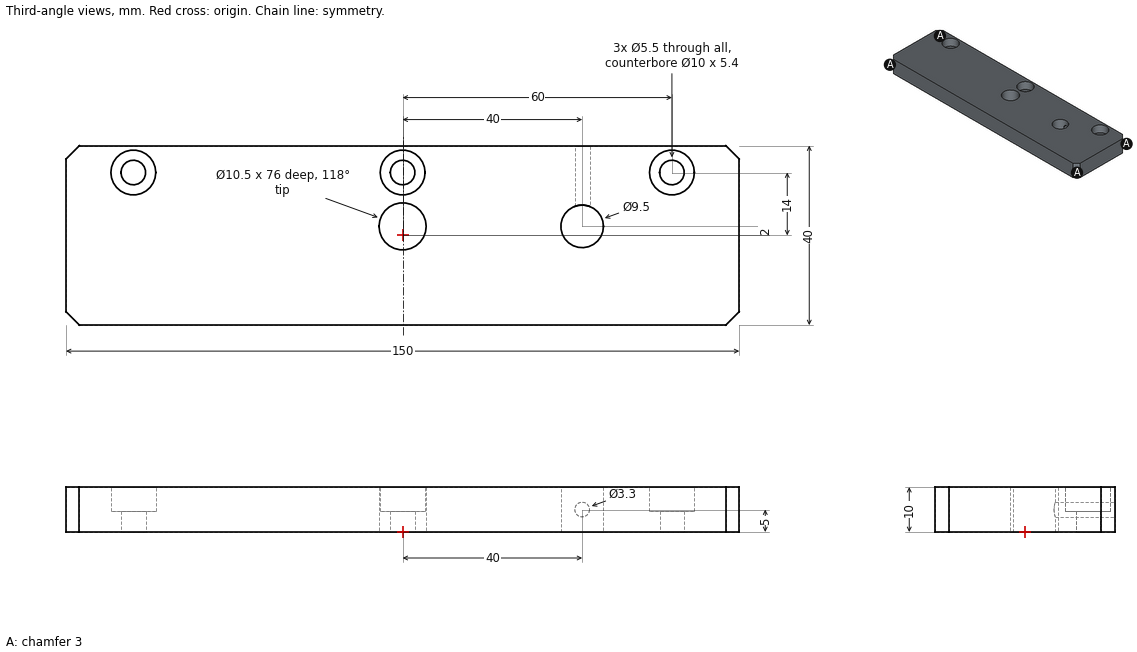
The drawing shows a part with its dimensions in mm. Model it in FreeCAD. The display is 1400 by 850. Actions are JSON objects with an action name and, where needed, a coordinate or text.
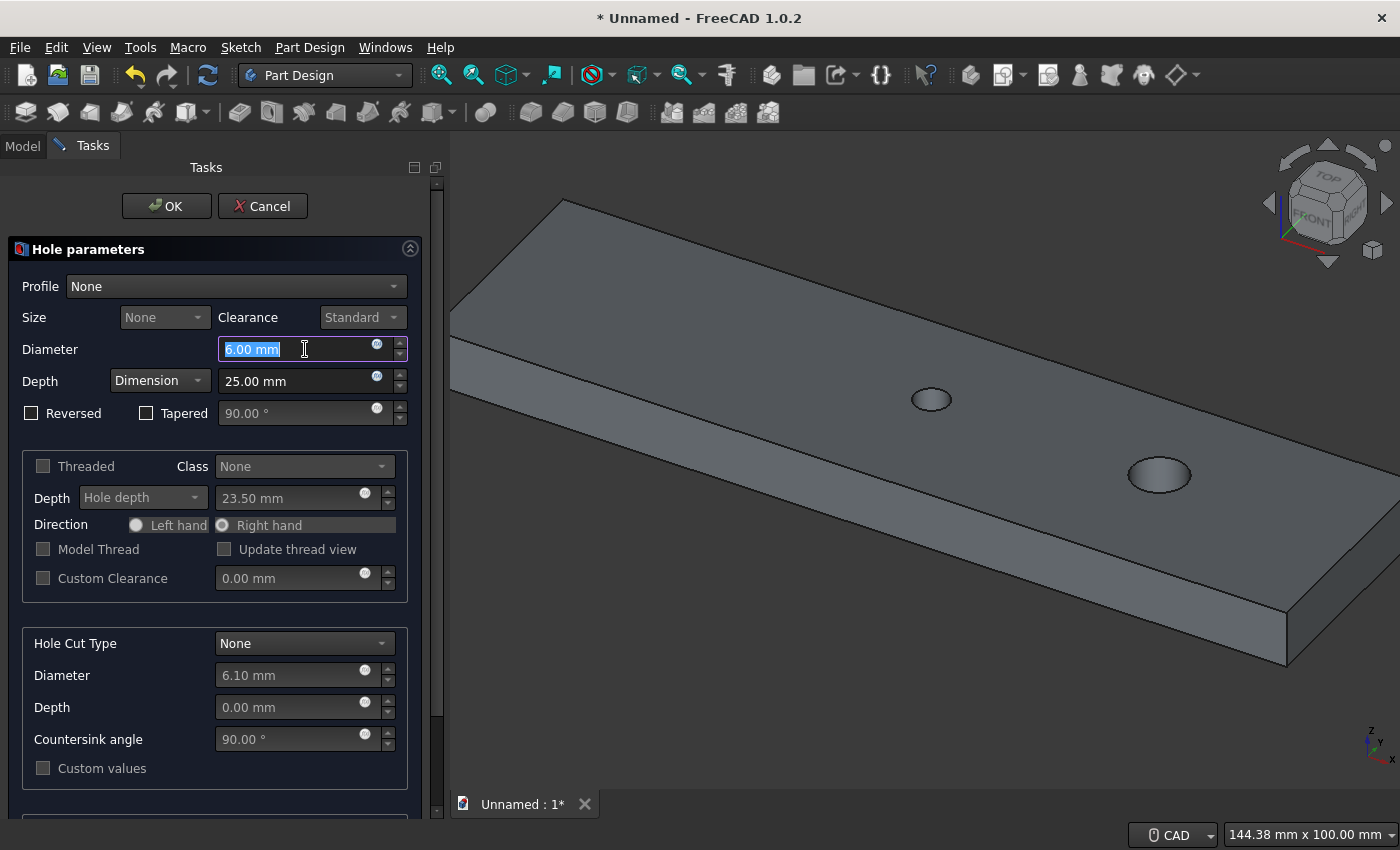
{"action": "type", "text": "10.5"}
{"action": "key", "text": "Tab"}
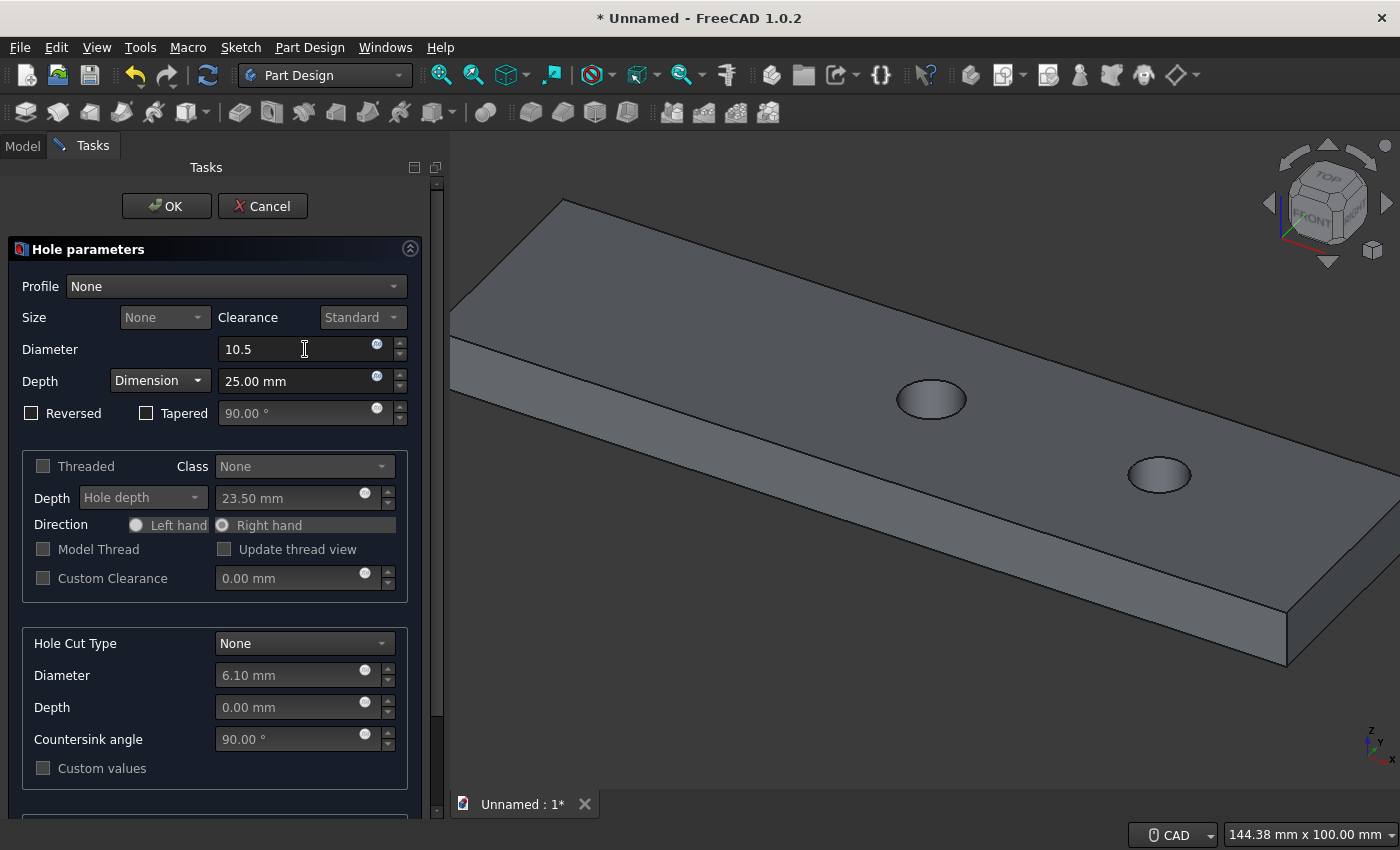
{"action": "triple_click", "coordinate": [305, 381]}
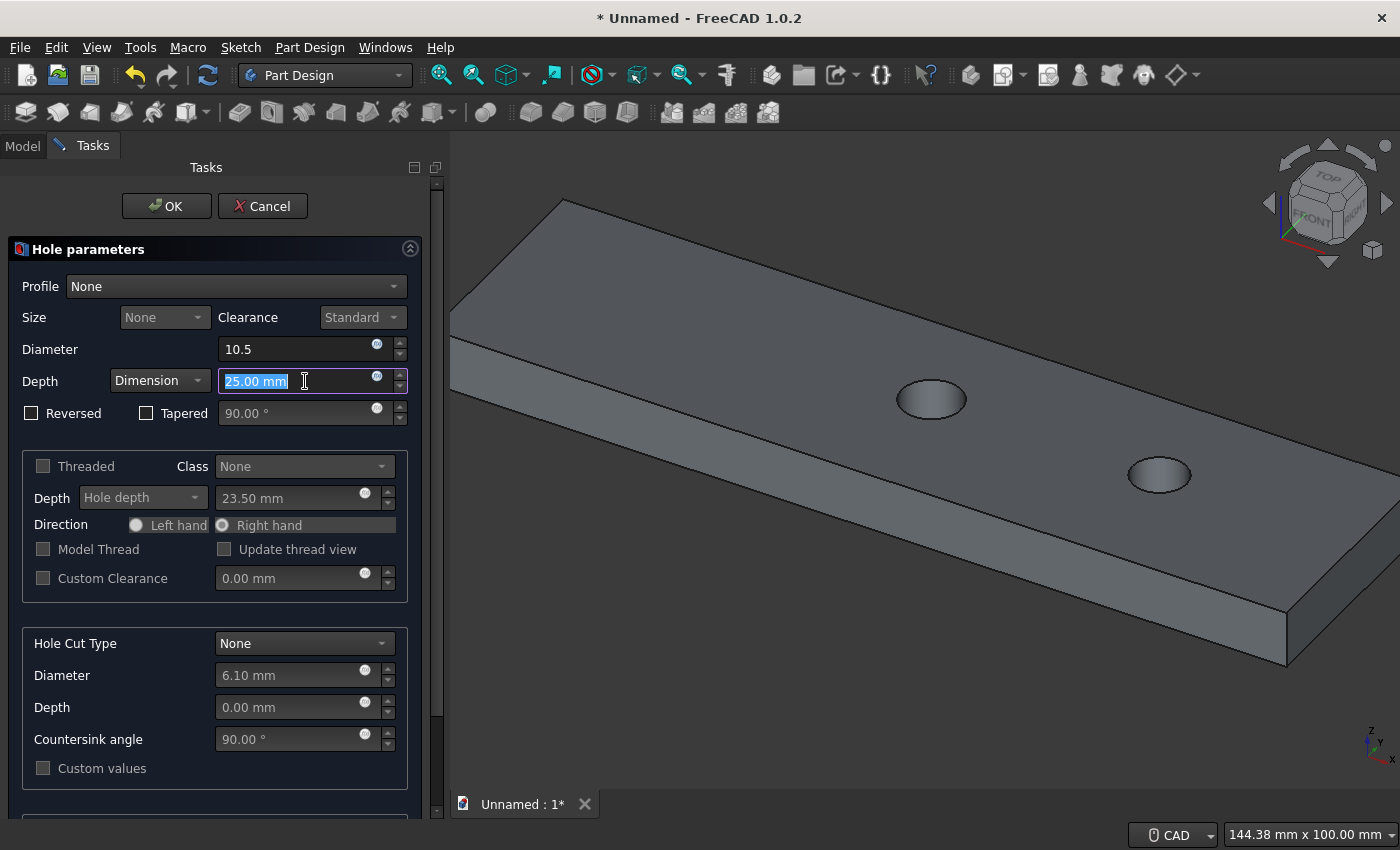
{"action": "type", "text": "76"}
{"action": "key", "text": "Tab"}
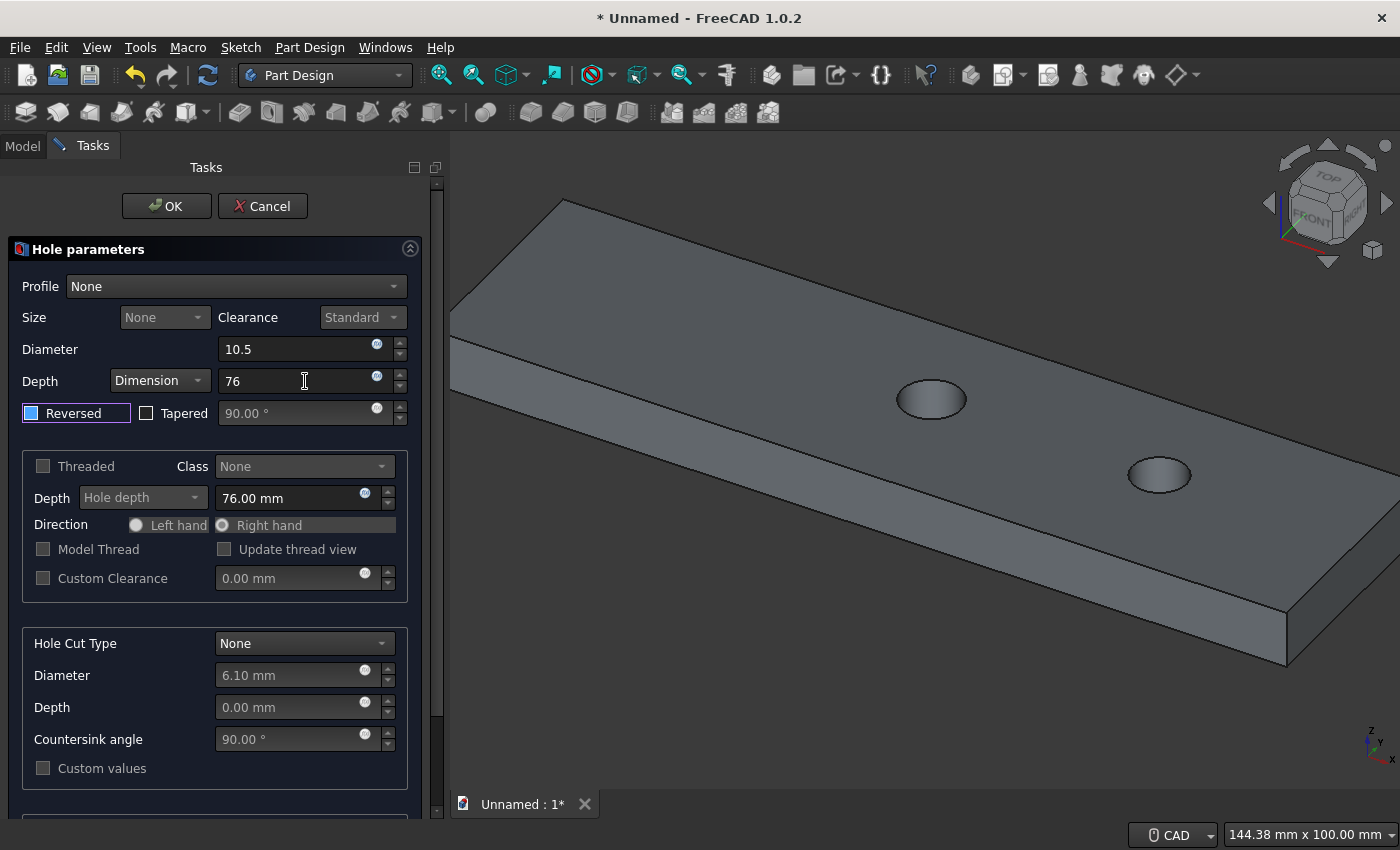
{"action": "left_click", "coordinate": [167, 206]}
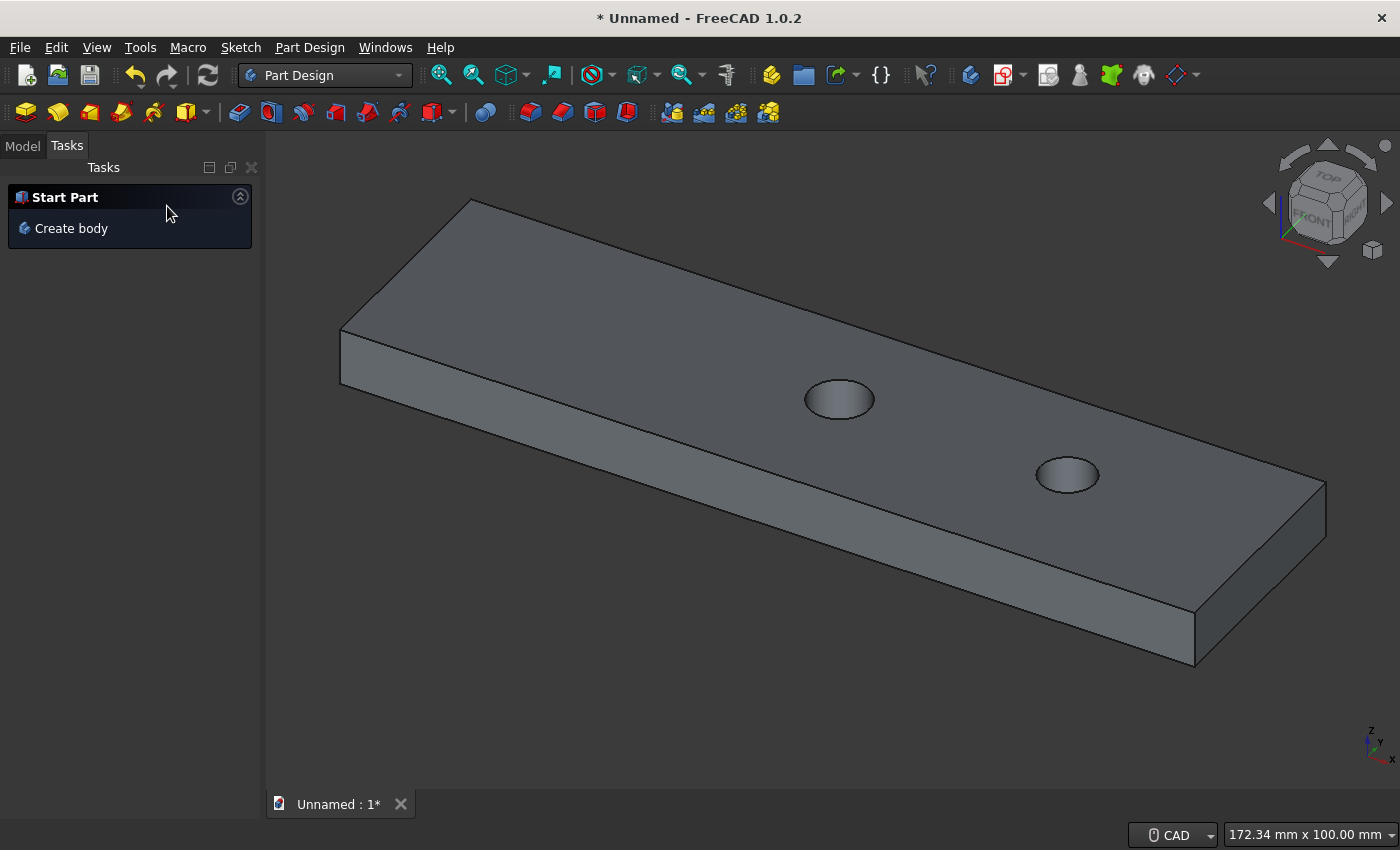
{"action": "left_click", "coordinate": [589, 324]}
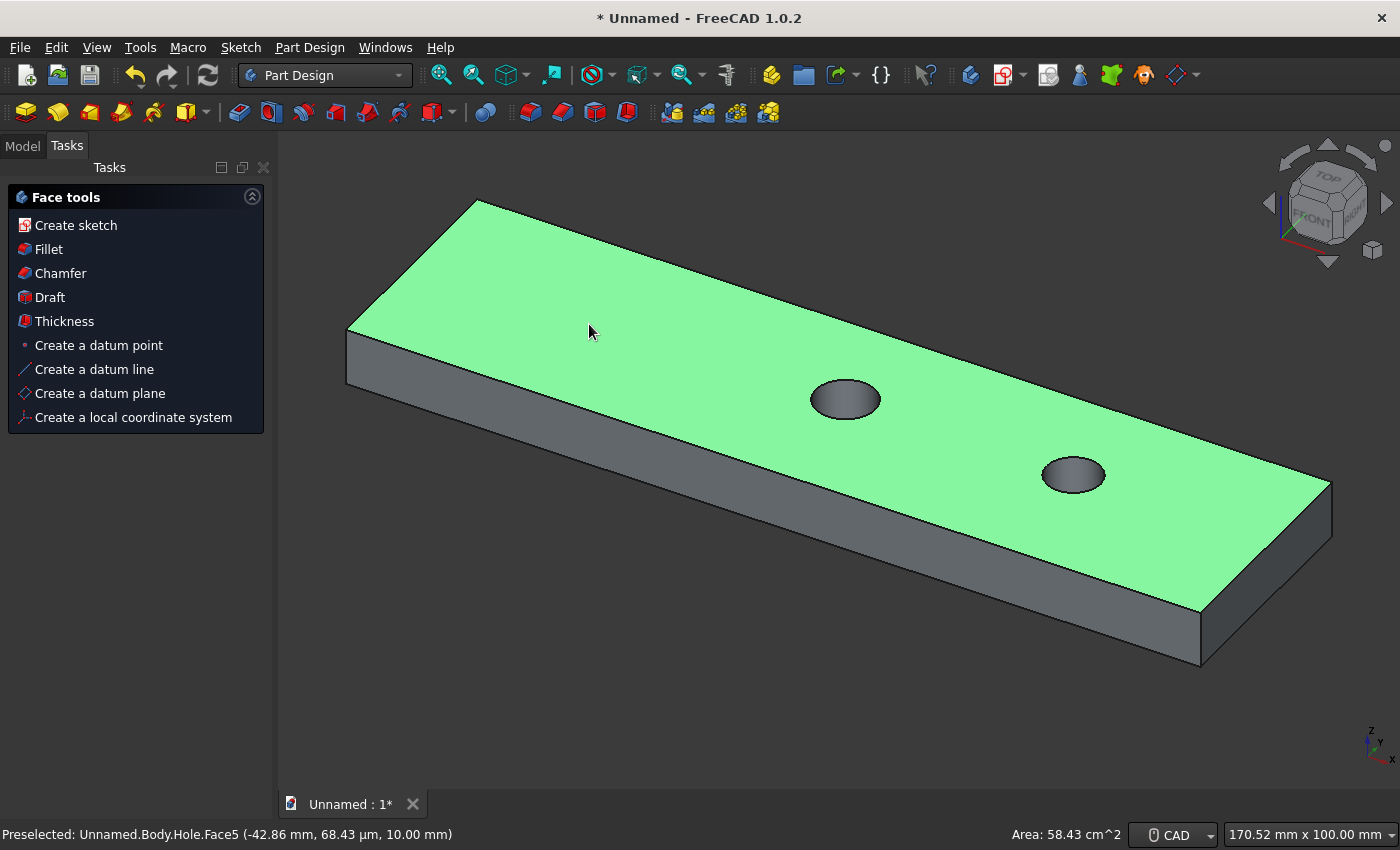
{"action": "left_click", "coordinate": [1004, 76]}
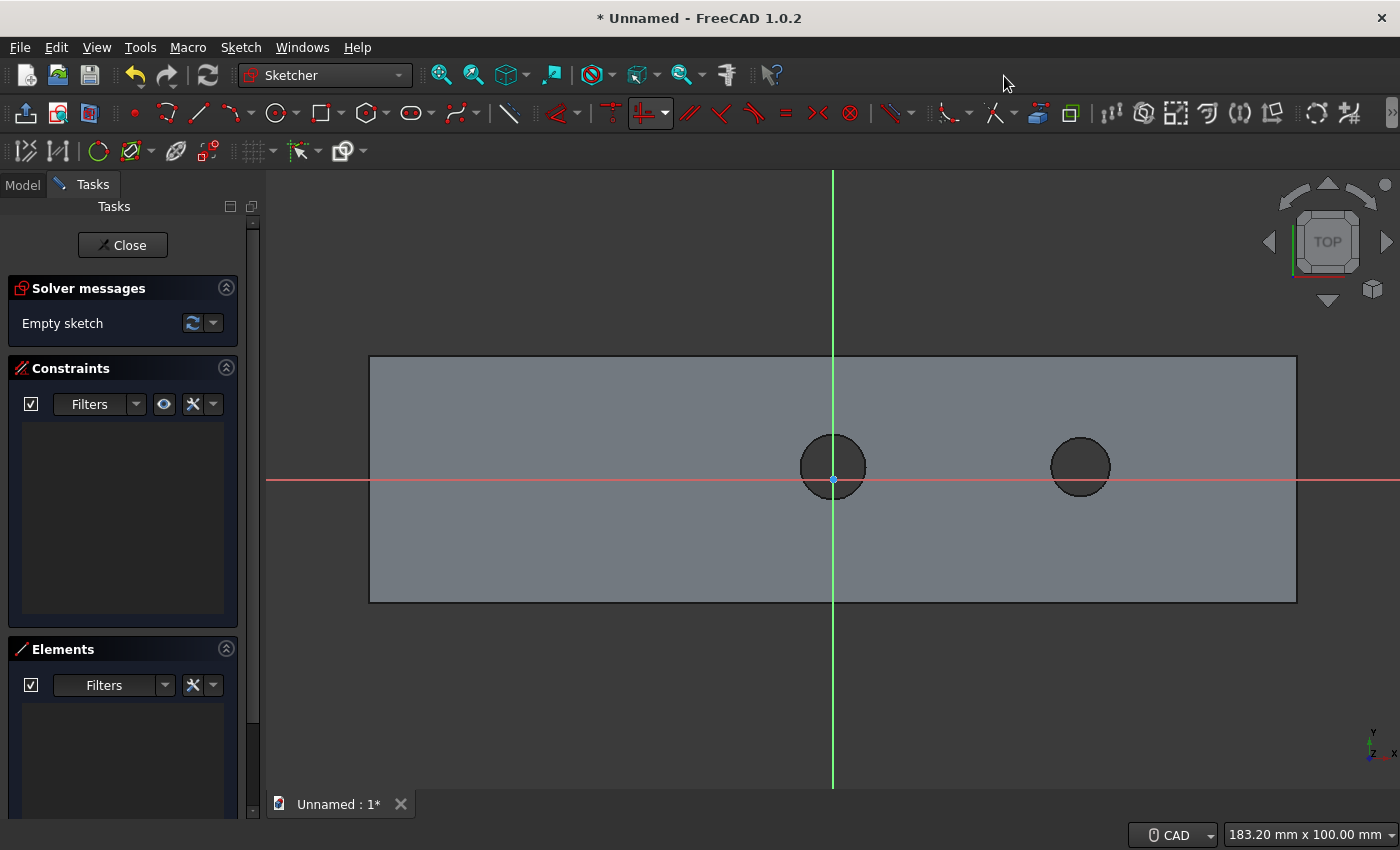
{"action": "scroll", "coordinate": [455, 714], "scroll_direction": "down", "scroll_amount": 1}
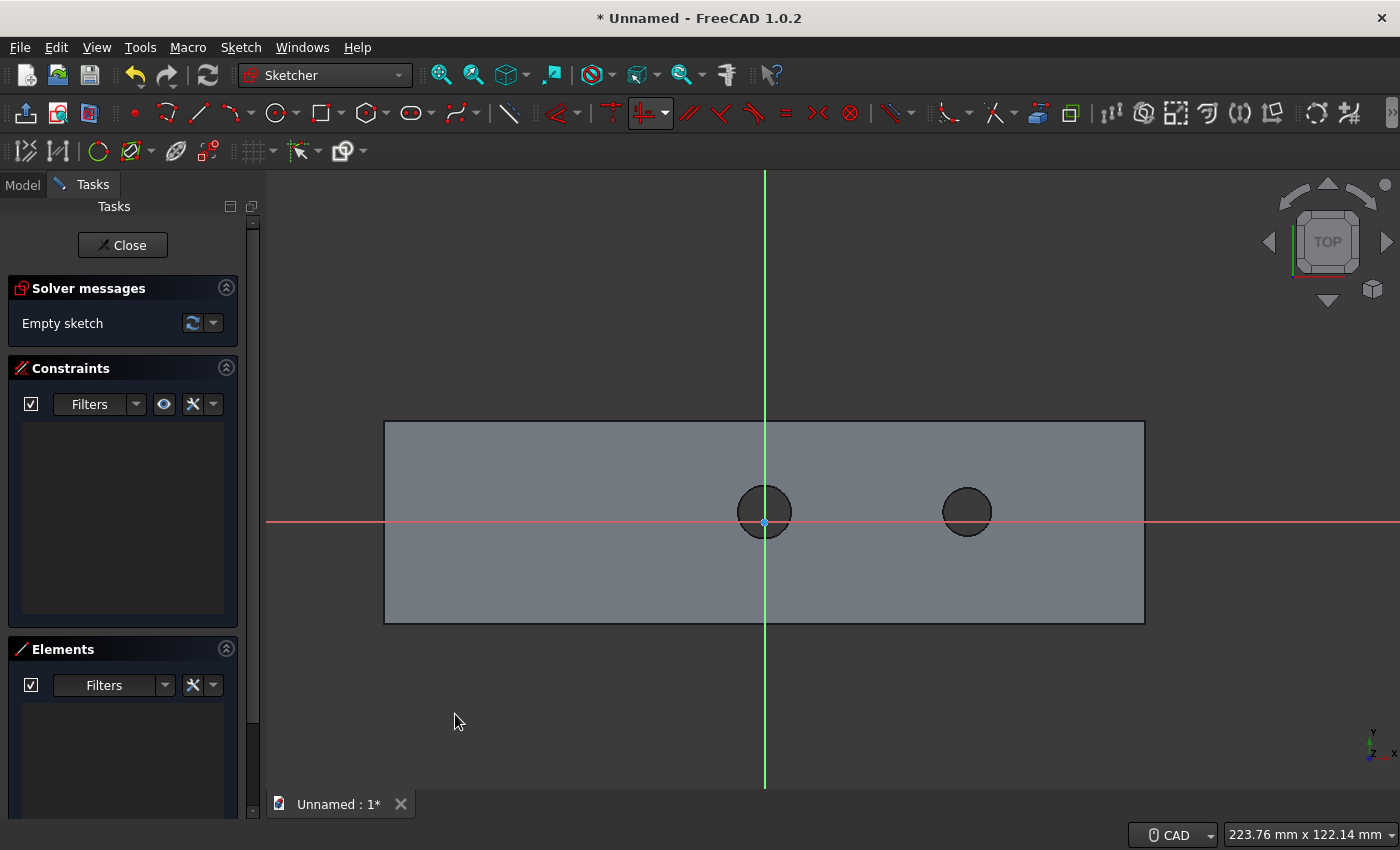
{"action": "key", "text": "g c"}